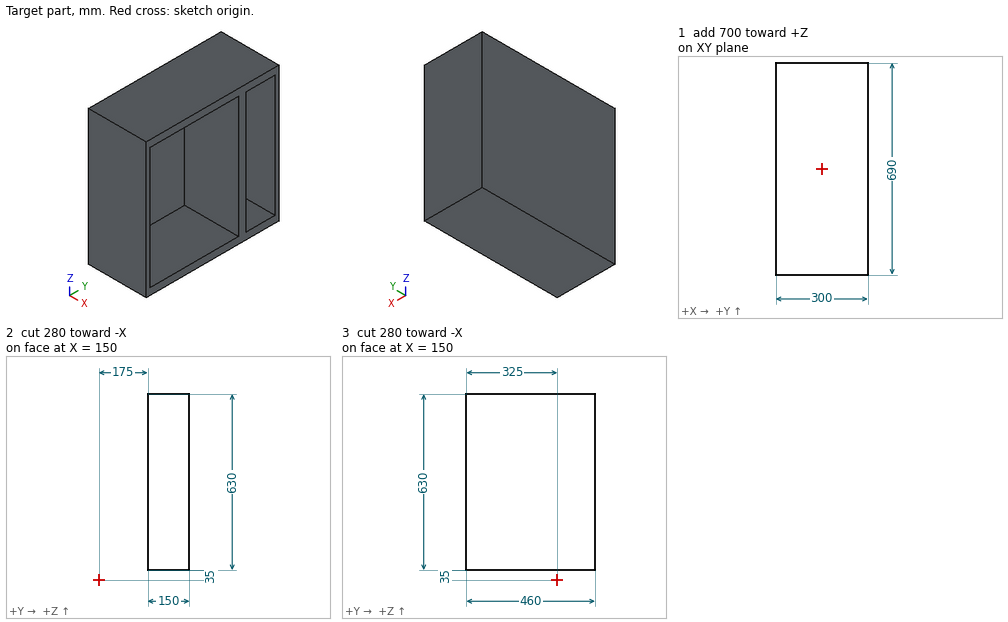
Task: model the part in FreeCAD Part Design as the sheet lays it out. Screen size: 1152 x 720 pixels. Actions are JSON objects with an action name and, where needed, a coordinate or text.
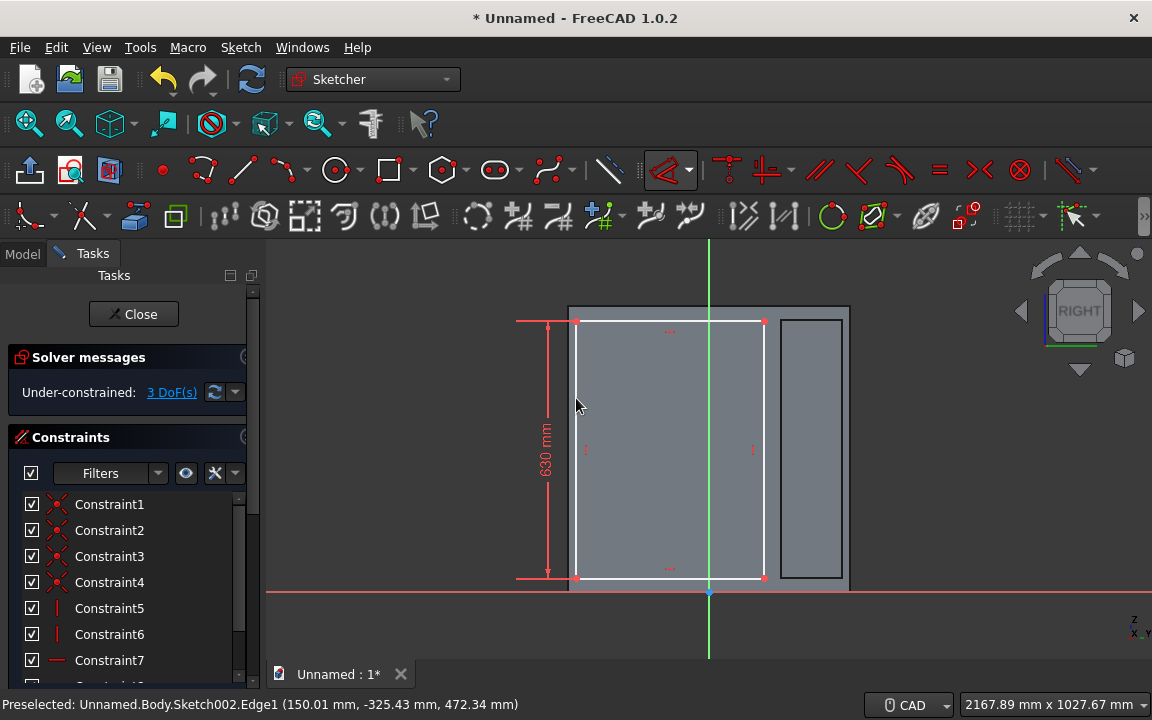
{"action": "left_click", "coordinate": [632, 579]}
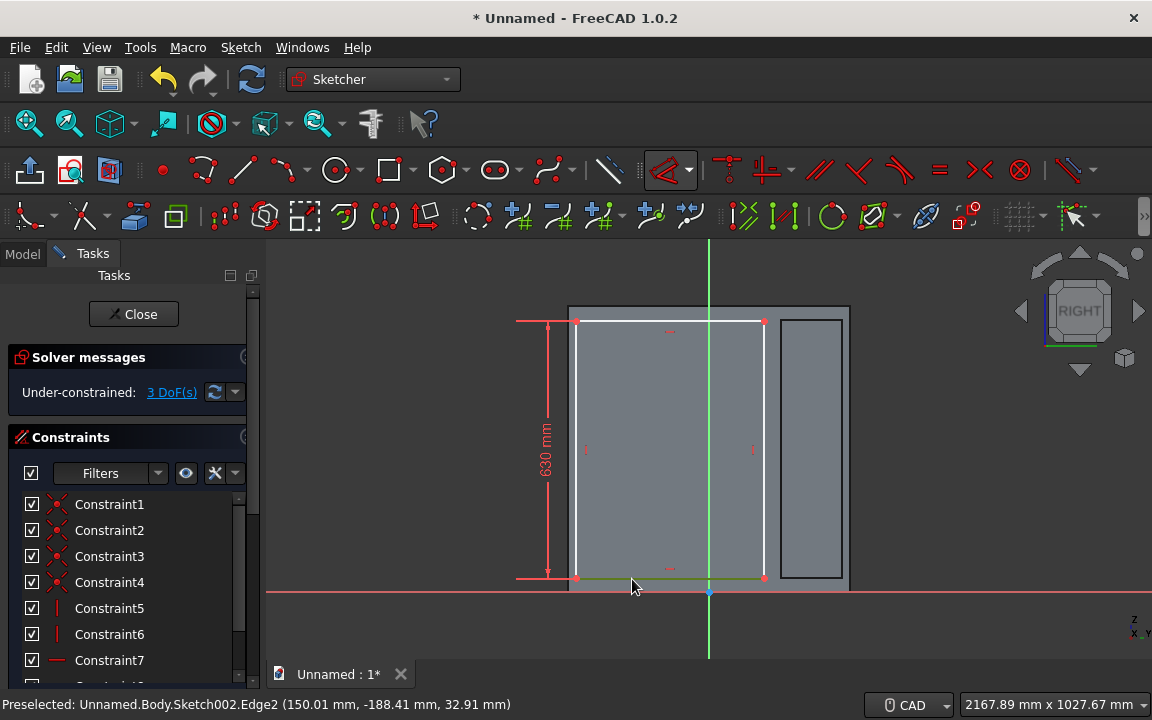
{"action": "key", "text": "l"}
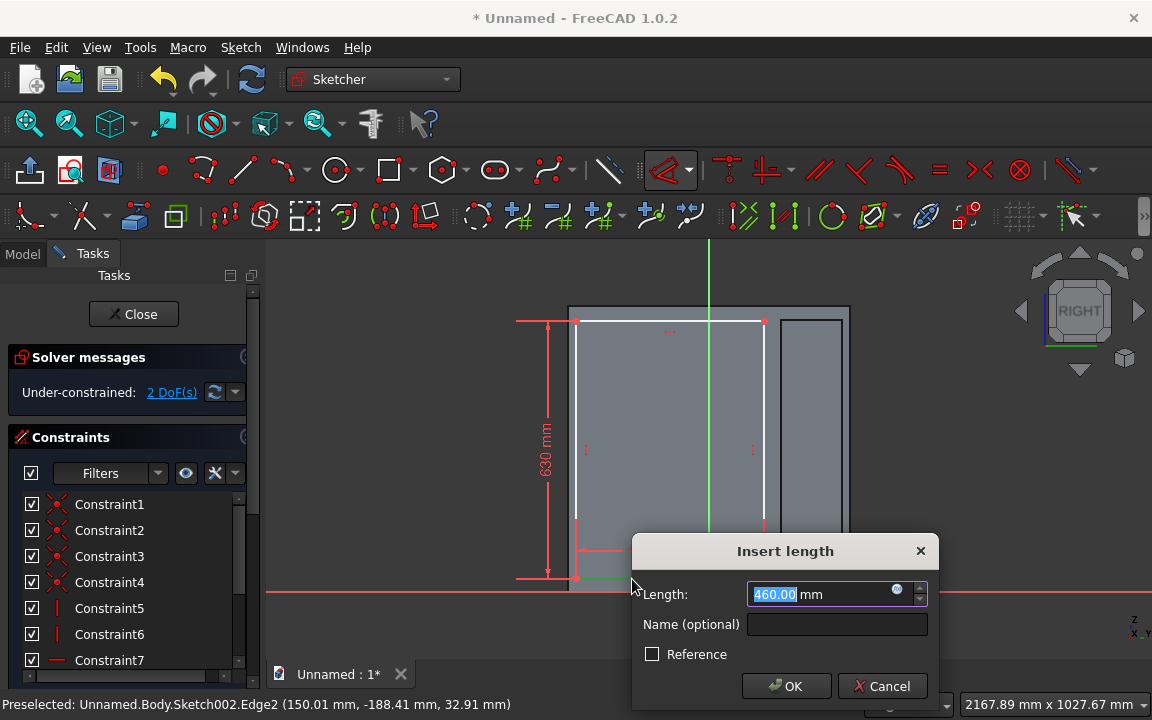
{"action": "type", "text": "460"}
{"action": "key", "text": "Return"}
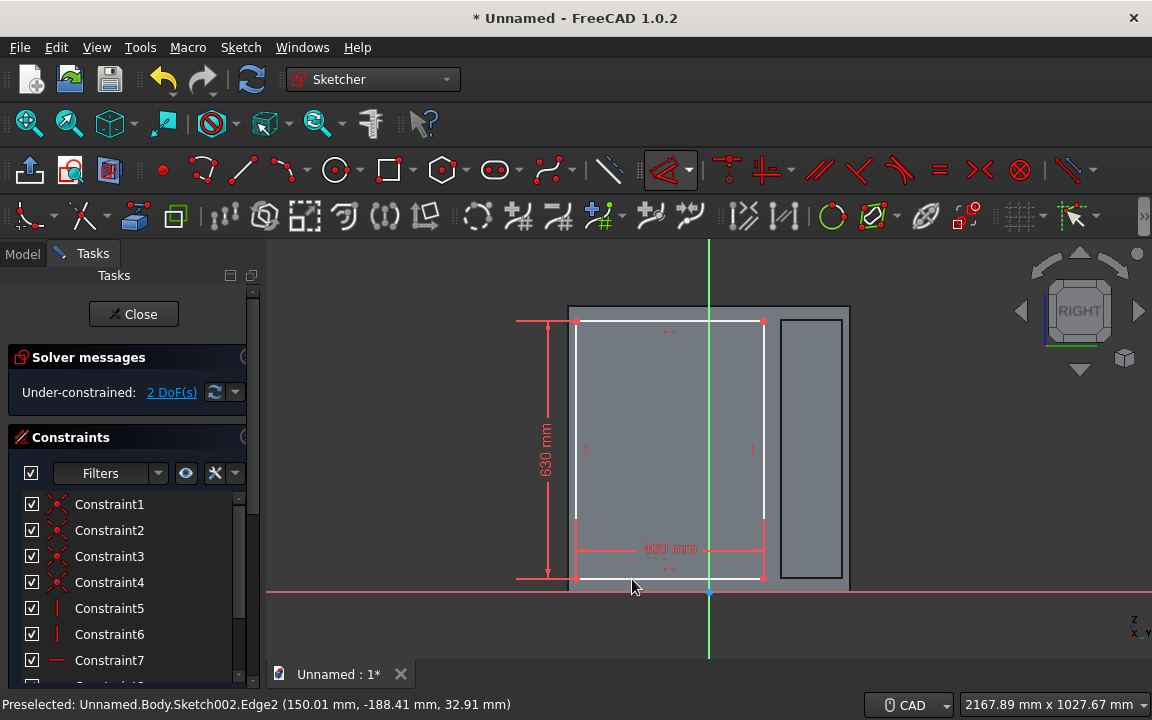
{"action": "scroll", "coordinate": [576, 579], "scroll_direction": "up", "scroll_amount": 6}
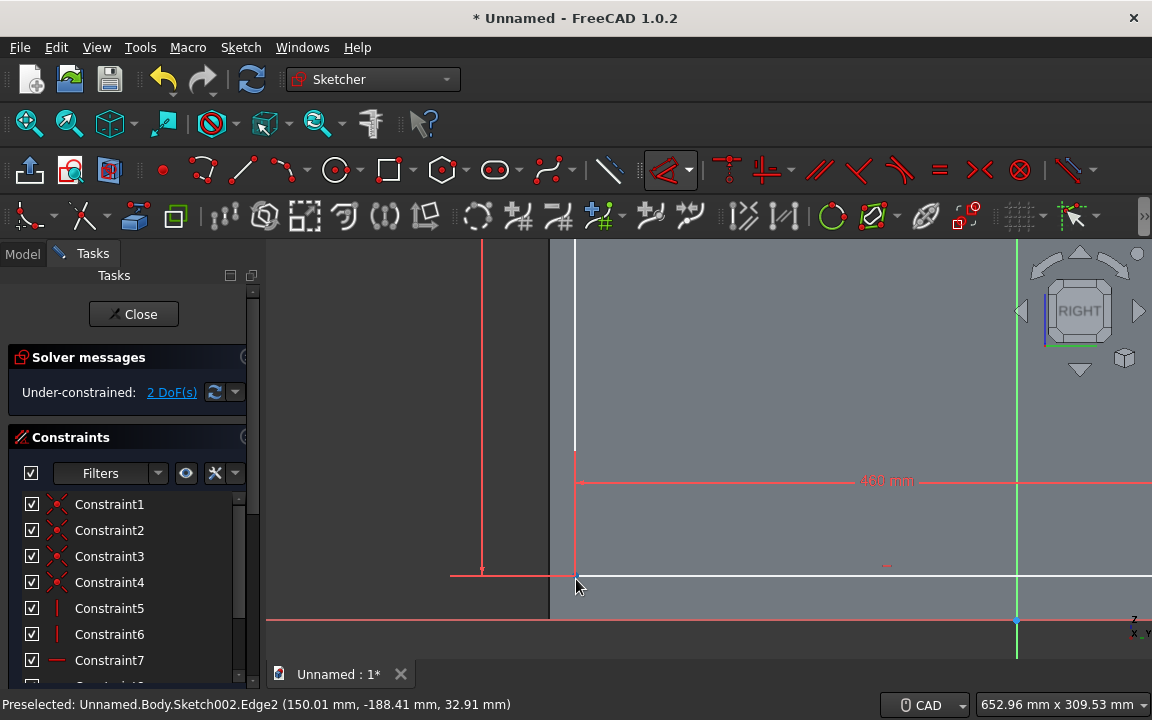
{"action": "left_click", "coordinate": [575, 576]}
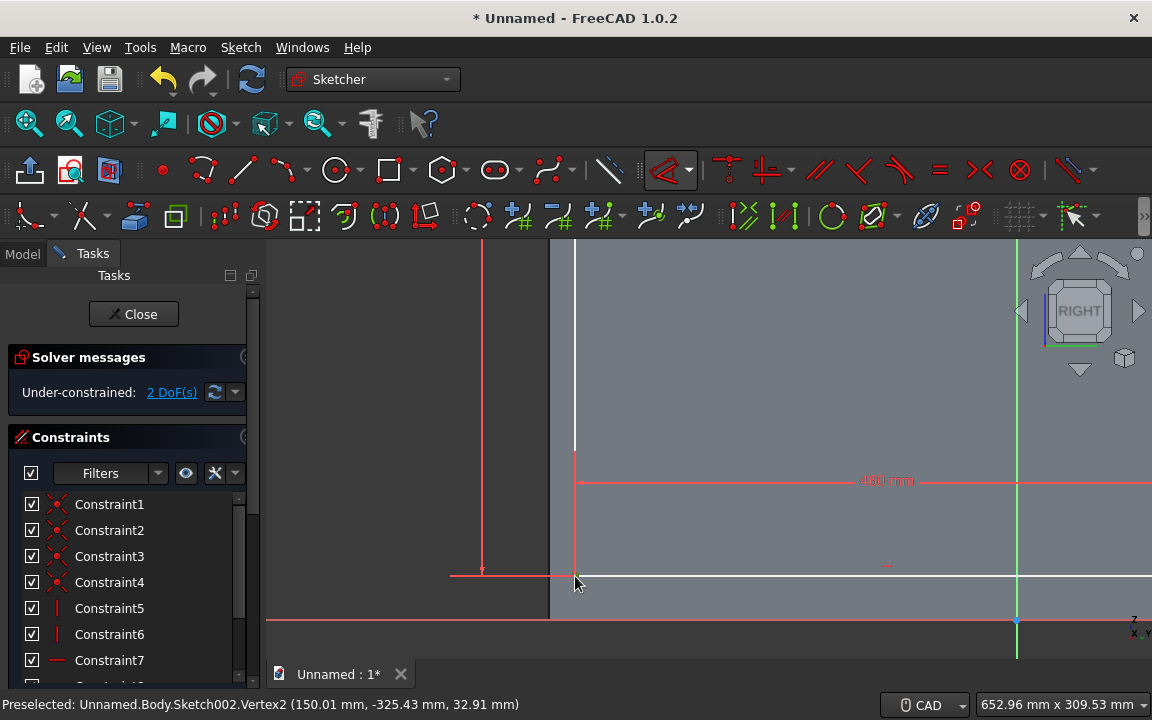
{"action": "left_click", "coordinate": [692, 170]}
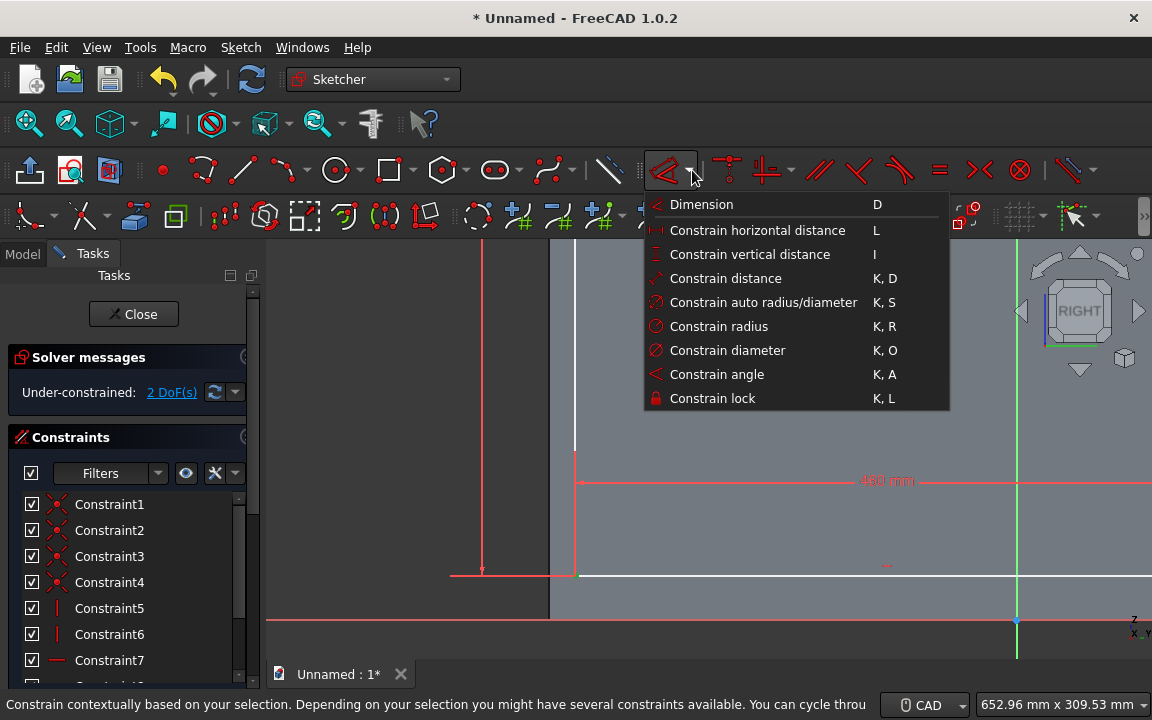
{"action": "left_click", "coordinate": [797, 254]}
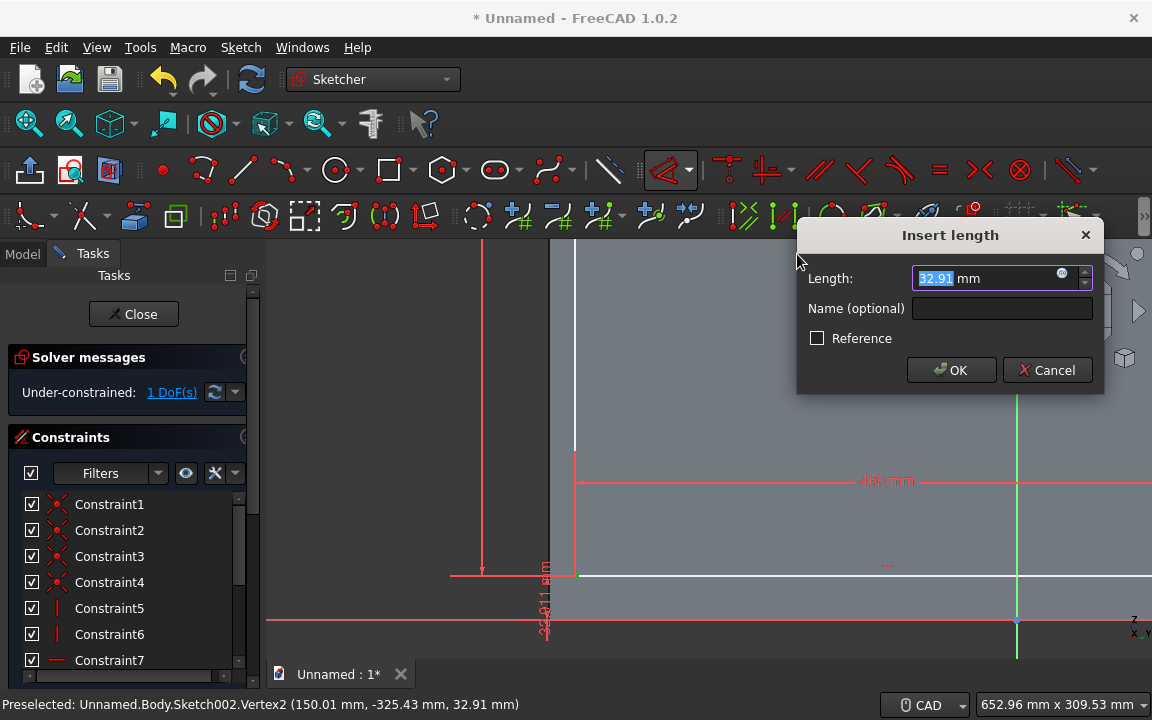
{"action": "type", "text": "35"}
{"action": "key", "text": "Return"}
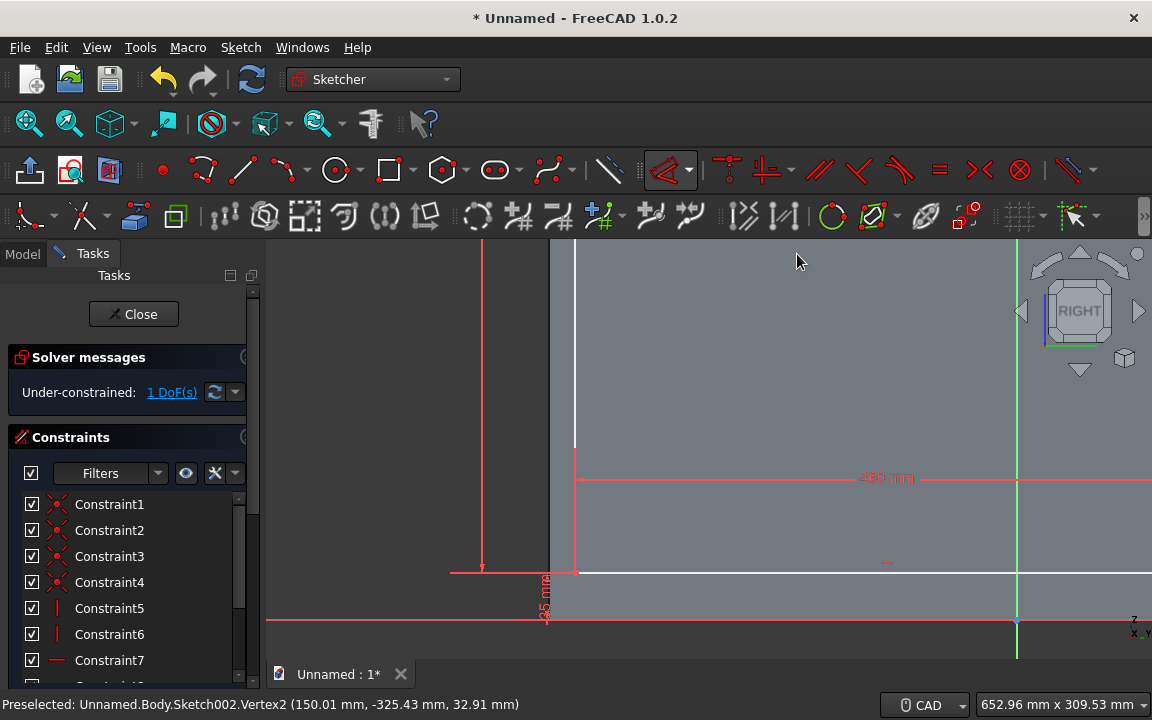
{"action": "scroll", "coordinate": [534, 570], "scroll_direction": "down", "scroll_amount": 6}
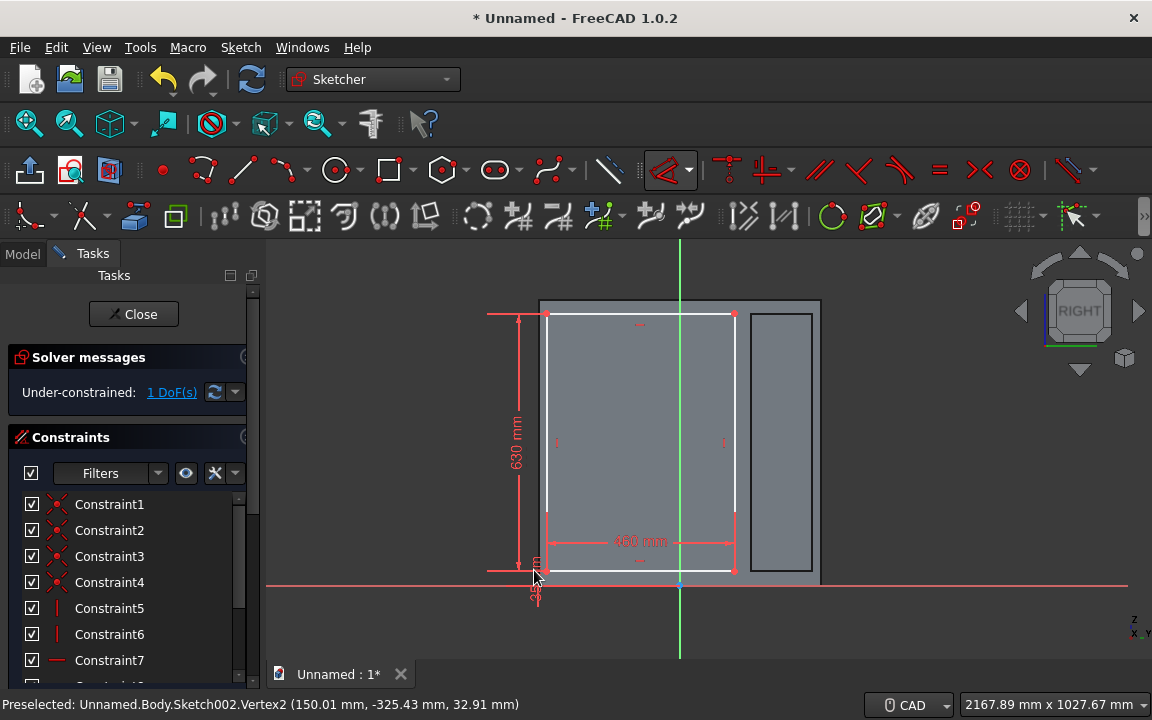
{"action": "left_click", "coordinate": [547, 314]}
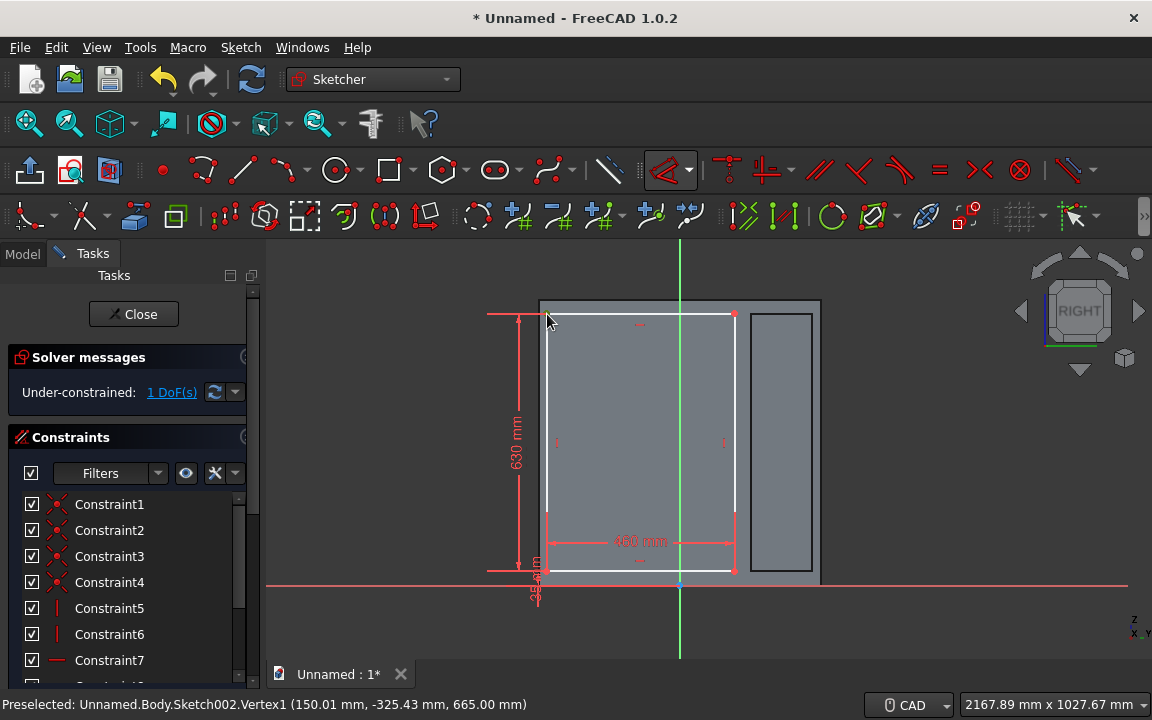
{"action": "left_click", "coordinate": [692, 170]}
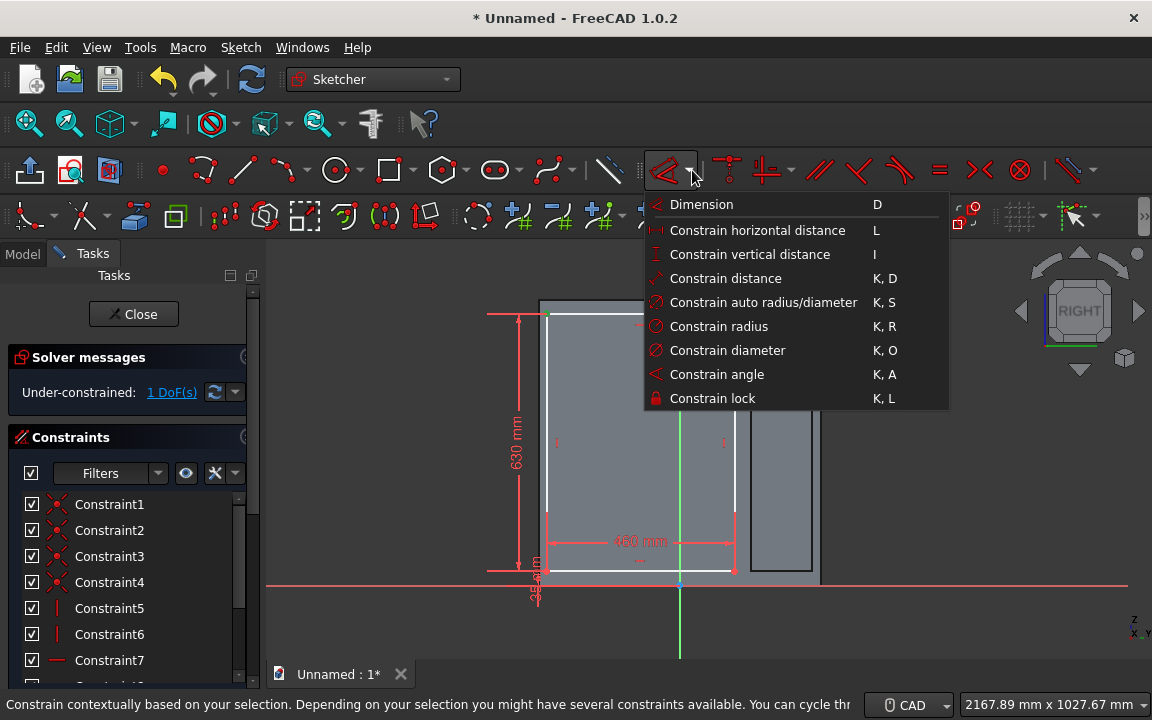
{"action": "left_click", "coordinate": [797, 230]}